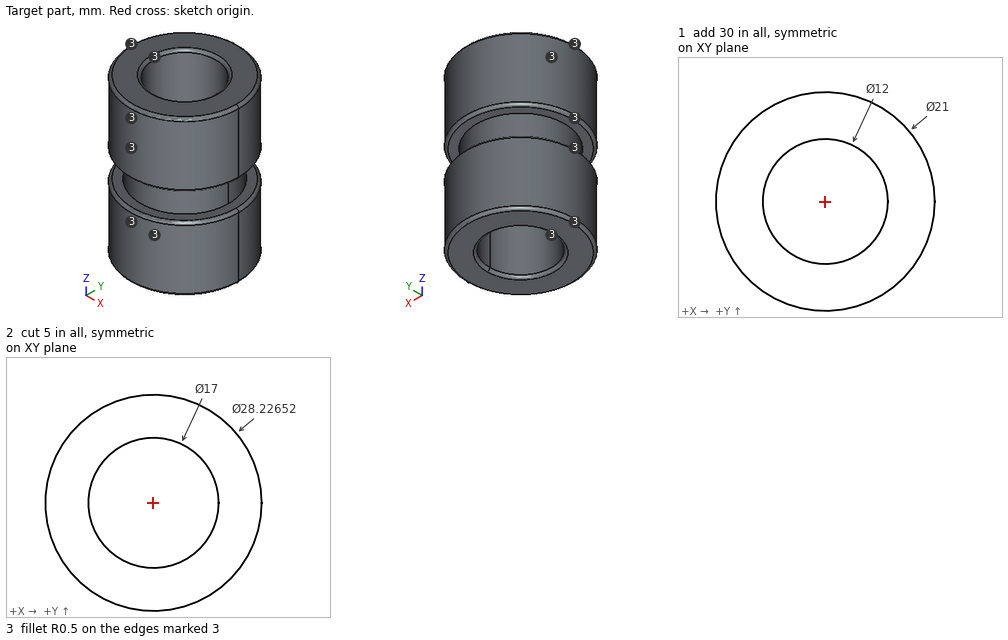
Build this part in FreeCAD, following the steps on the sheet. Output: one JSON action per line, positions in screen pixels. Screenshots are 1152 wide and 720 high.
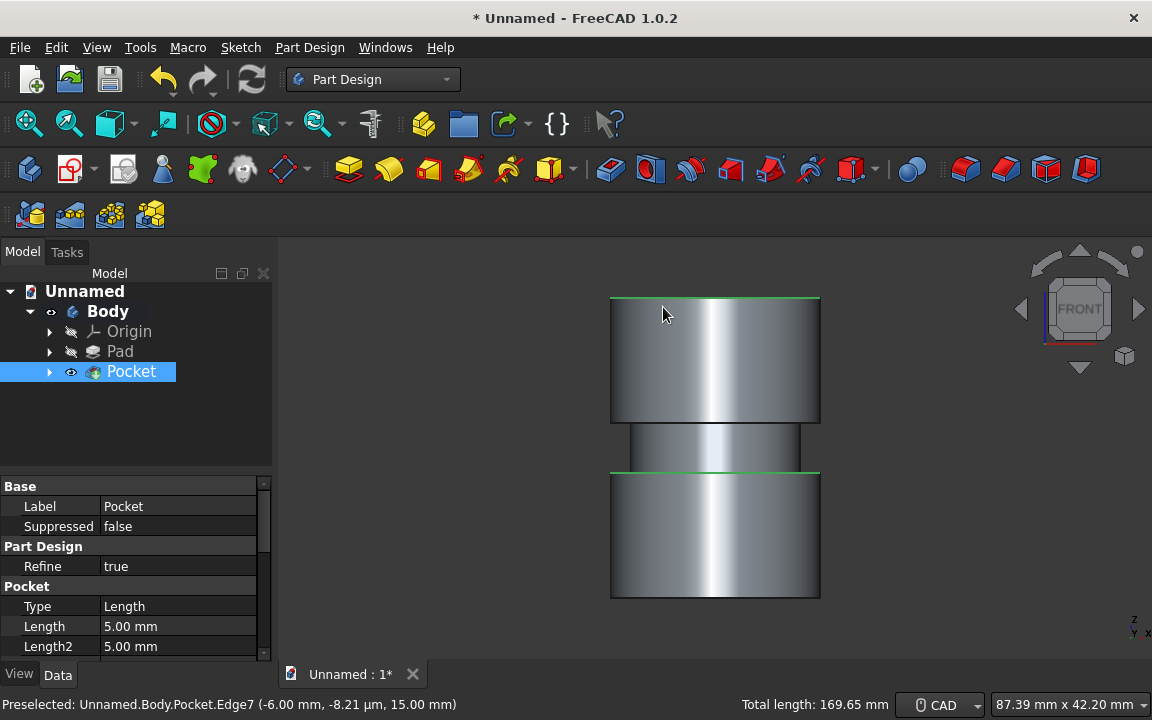
{"action": "left_click", "coordinate": [630, 422], "text": "ctrl"}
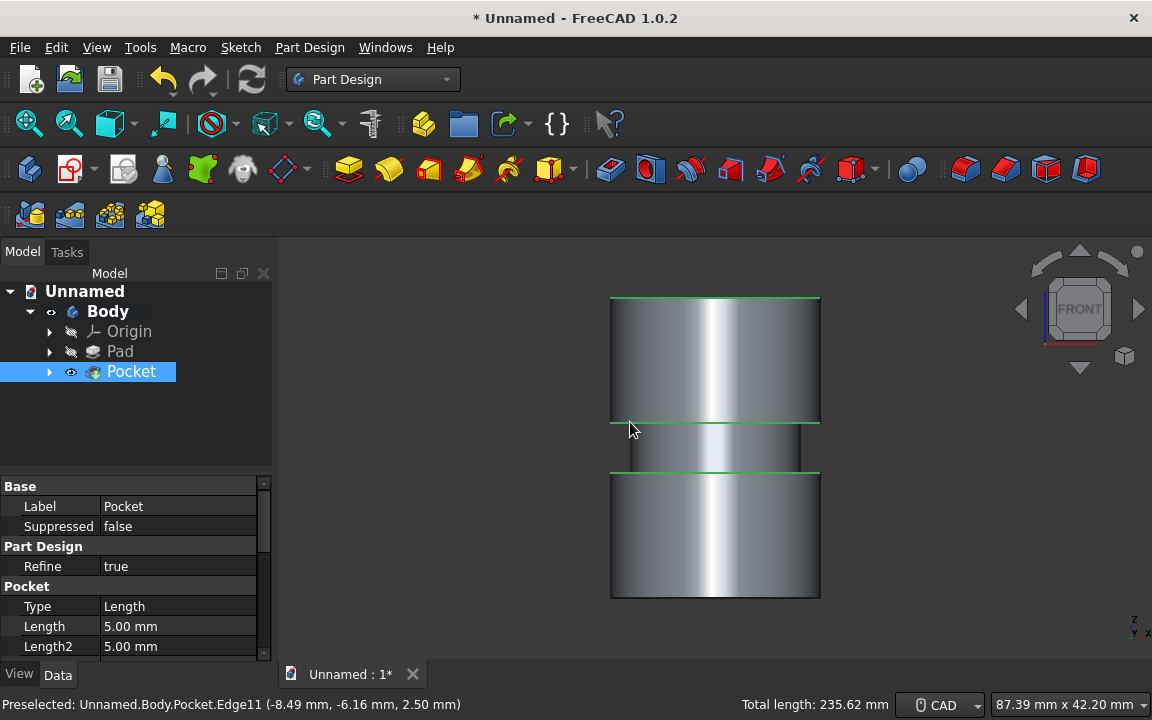
{"action": "left_click", "coordinate": [630, 597], "text": "ctrl"}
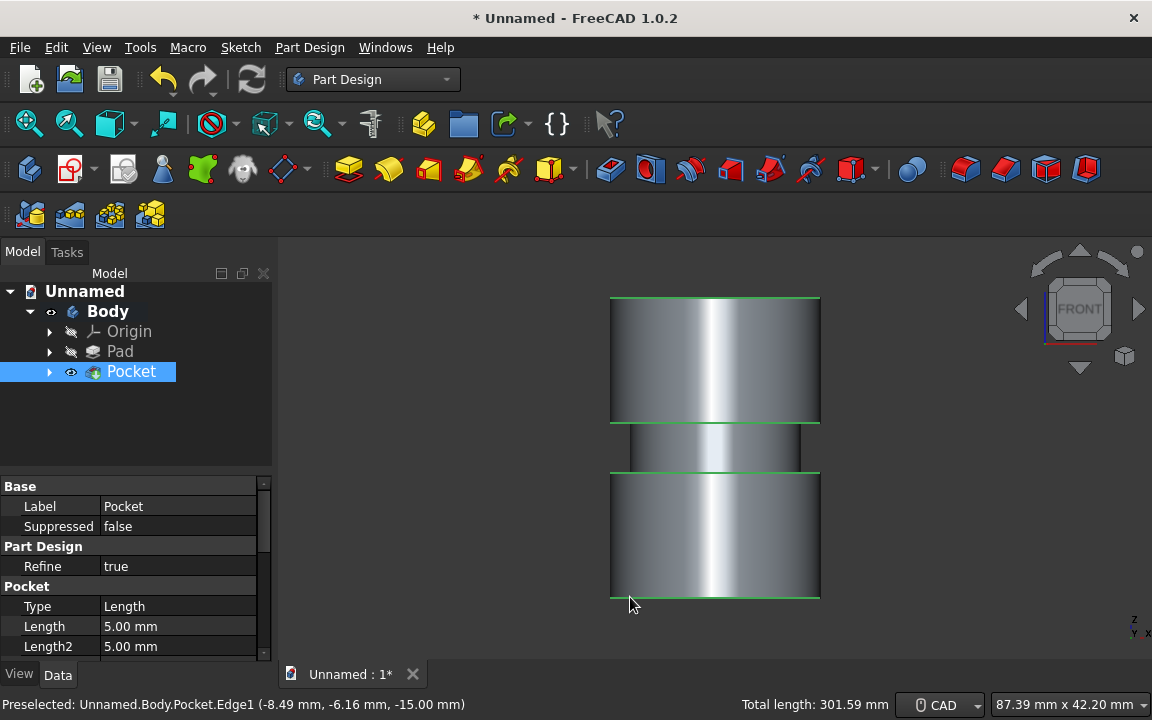
{"action": "key", "text": "3"}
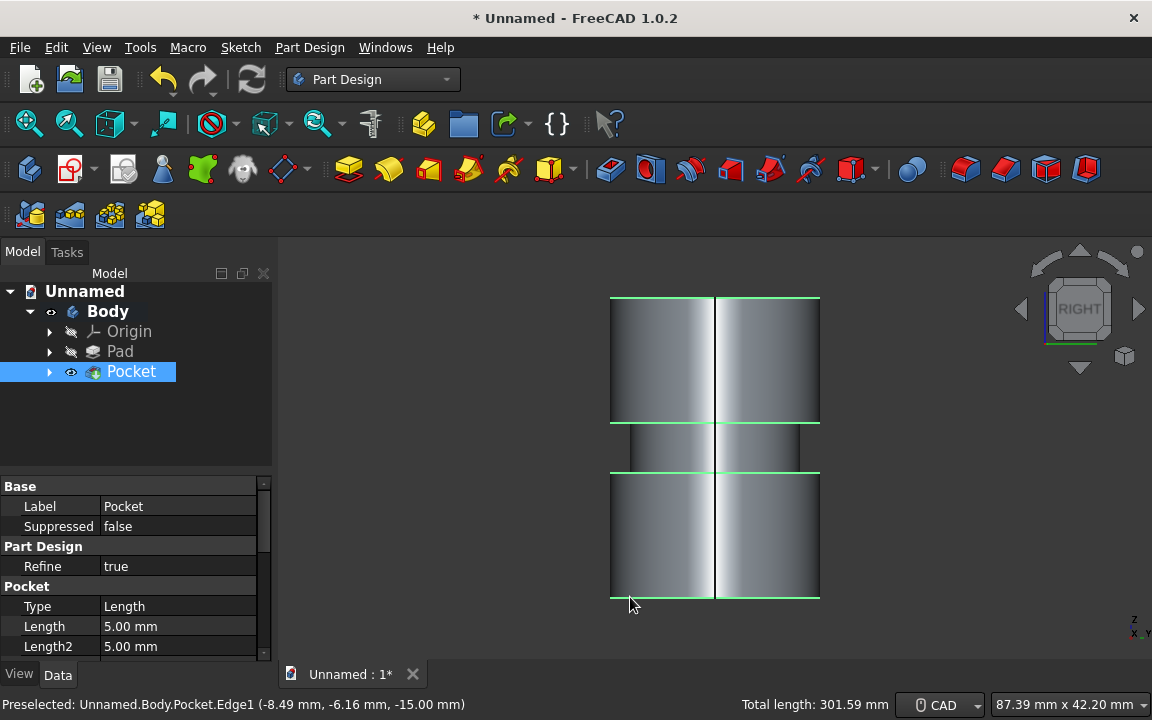
{"action": "key", "text": "5"}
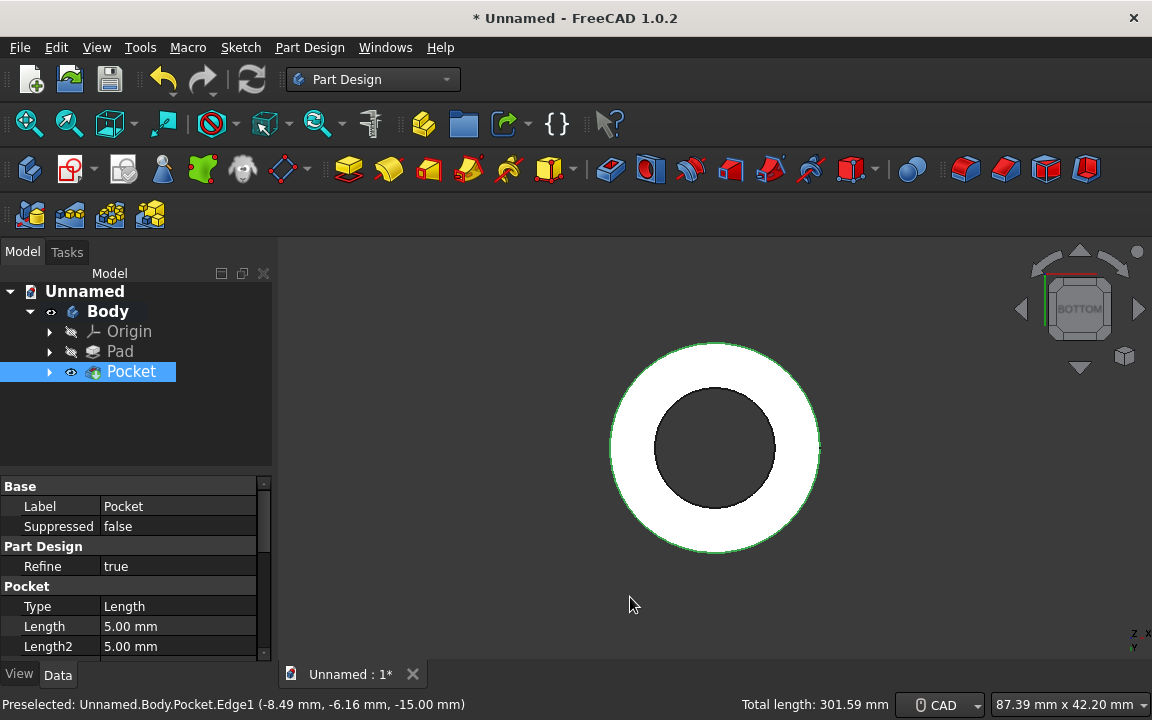
{"action": "left_click", "coordinate": [655, 447], "text": "ctrl"}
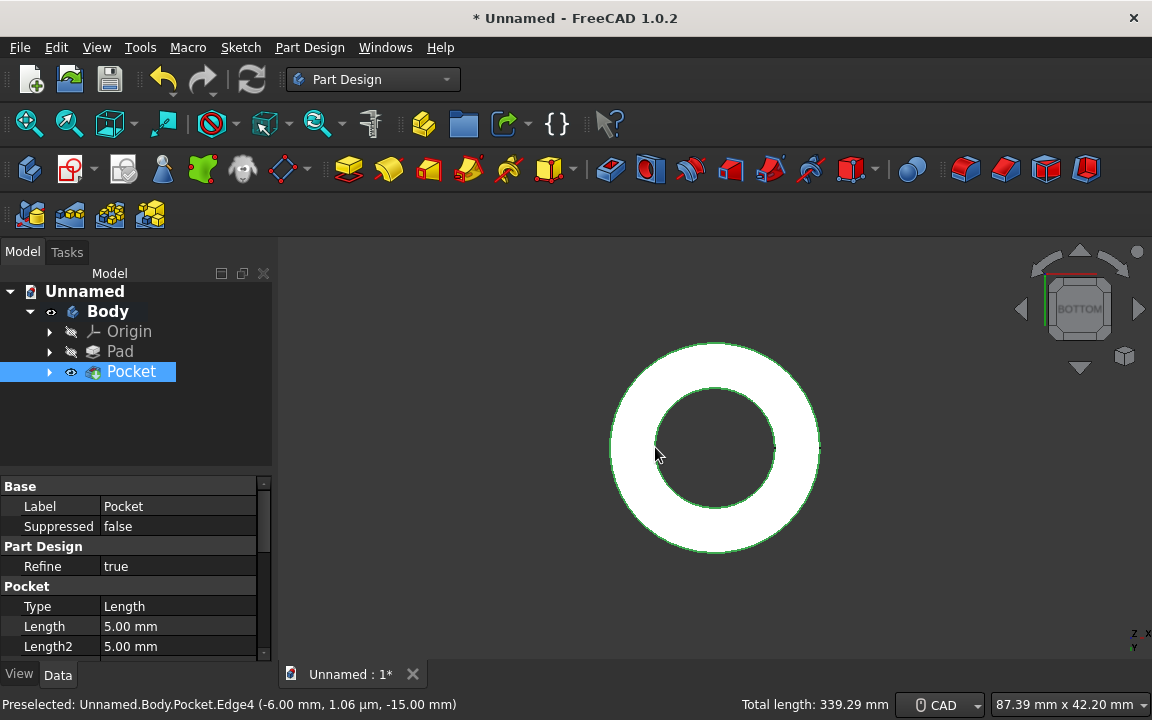
{"action": "left_click", "coordinate": [966, 170]}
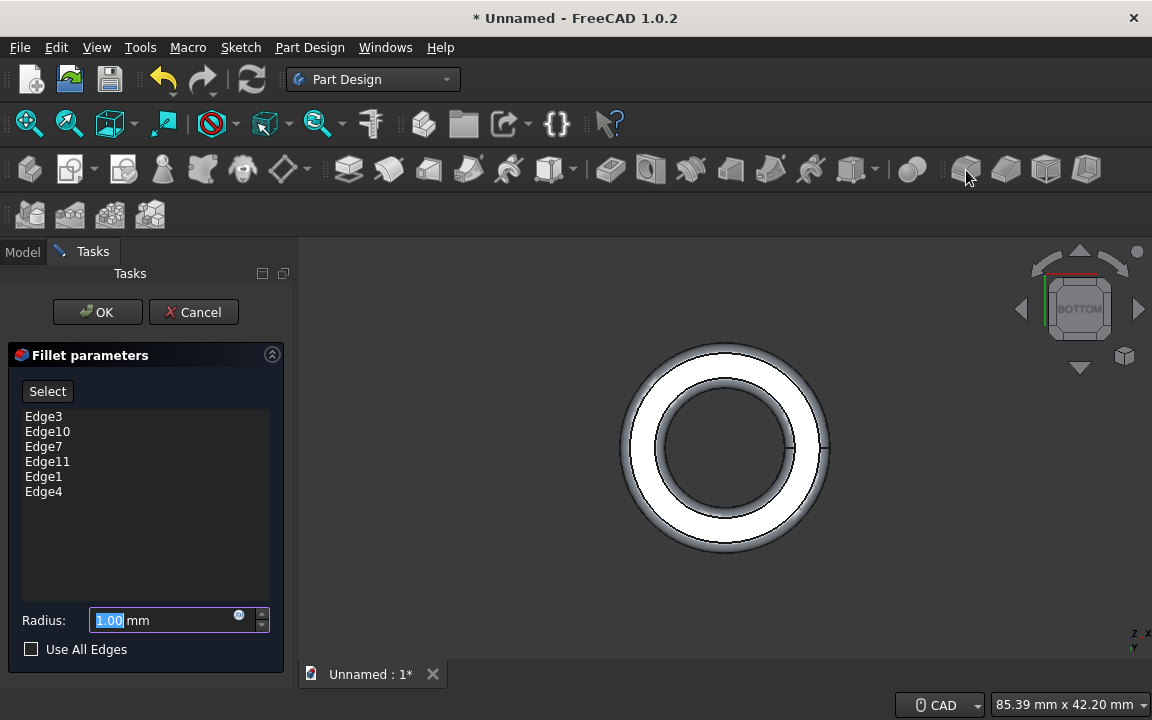
{"action": "type", "text": "0.5"}
{"action": "key", "text": "Tab"}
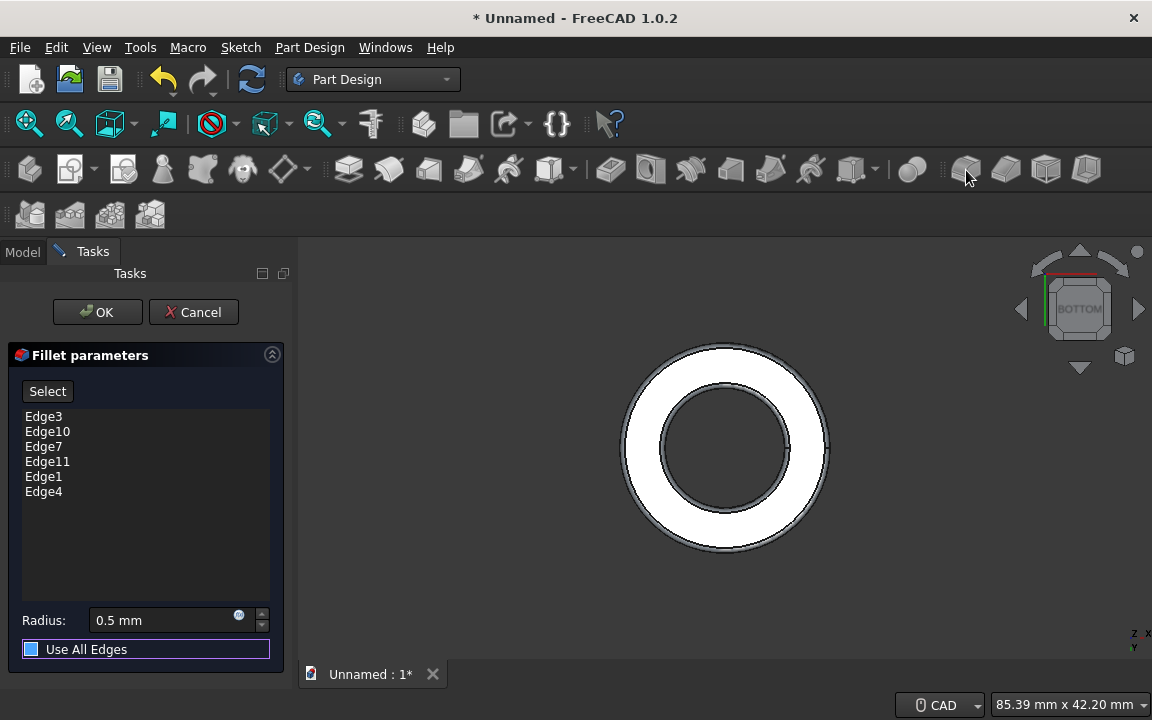
{"action": "left_click", "coordinate": [98, 312]}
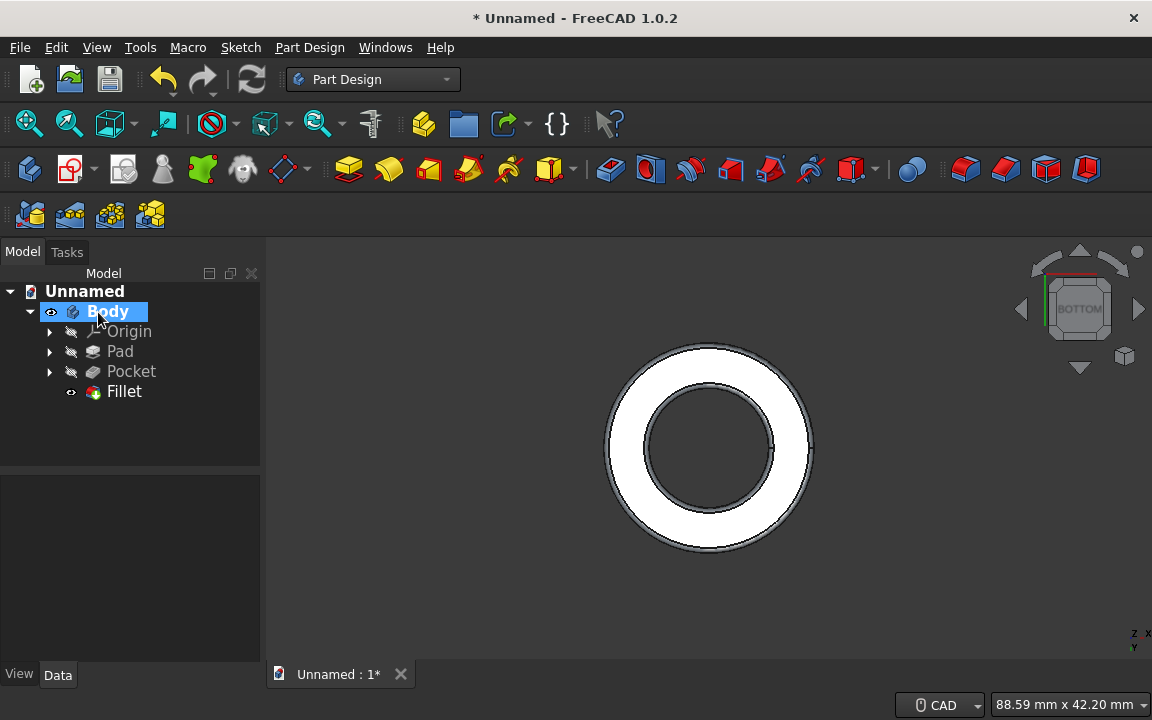
{"action": "key", "text": "0"}